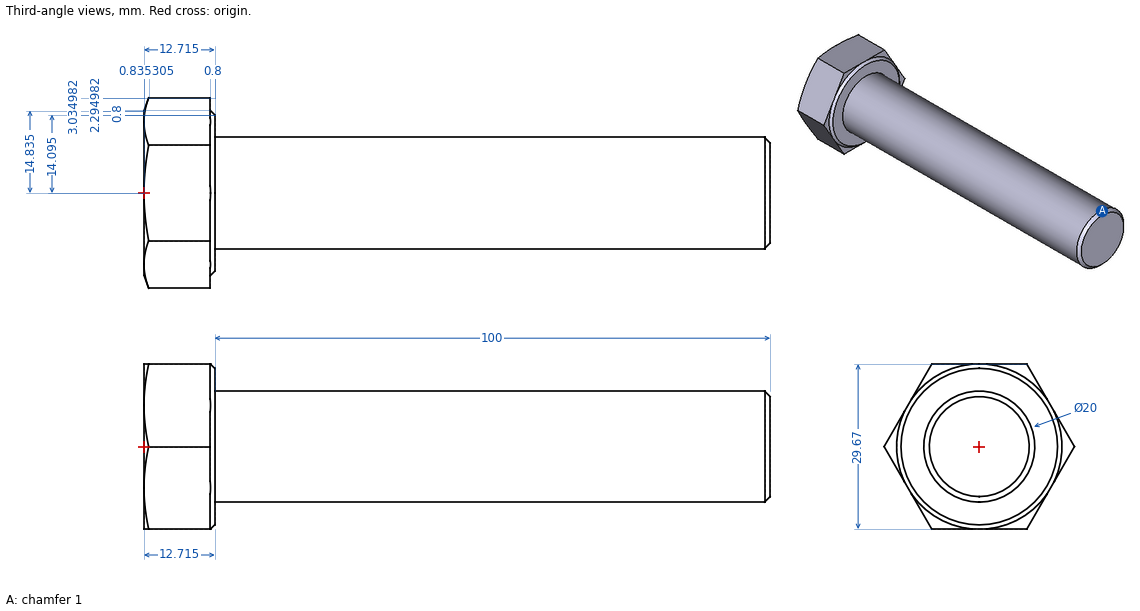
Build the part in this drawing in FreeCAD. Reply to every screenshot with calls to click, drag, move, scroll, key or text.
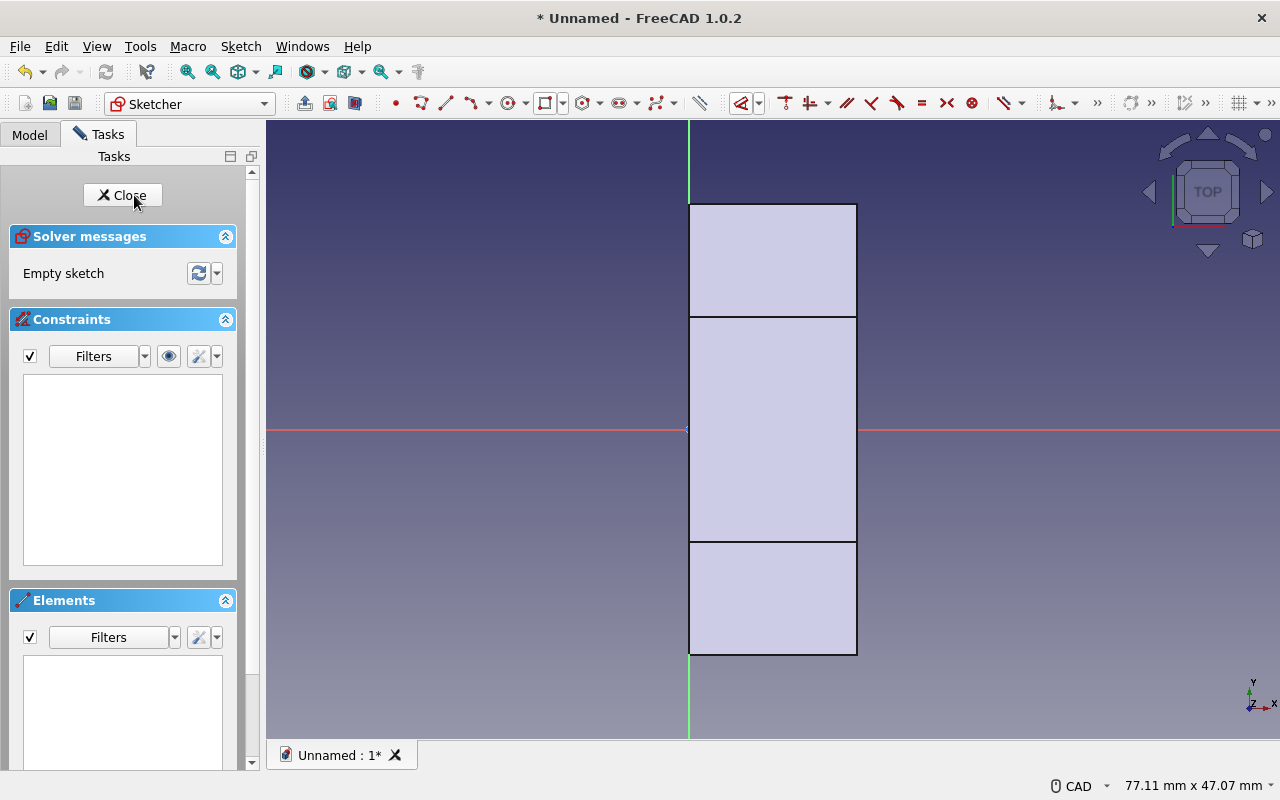
key(q)
key(s)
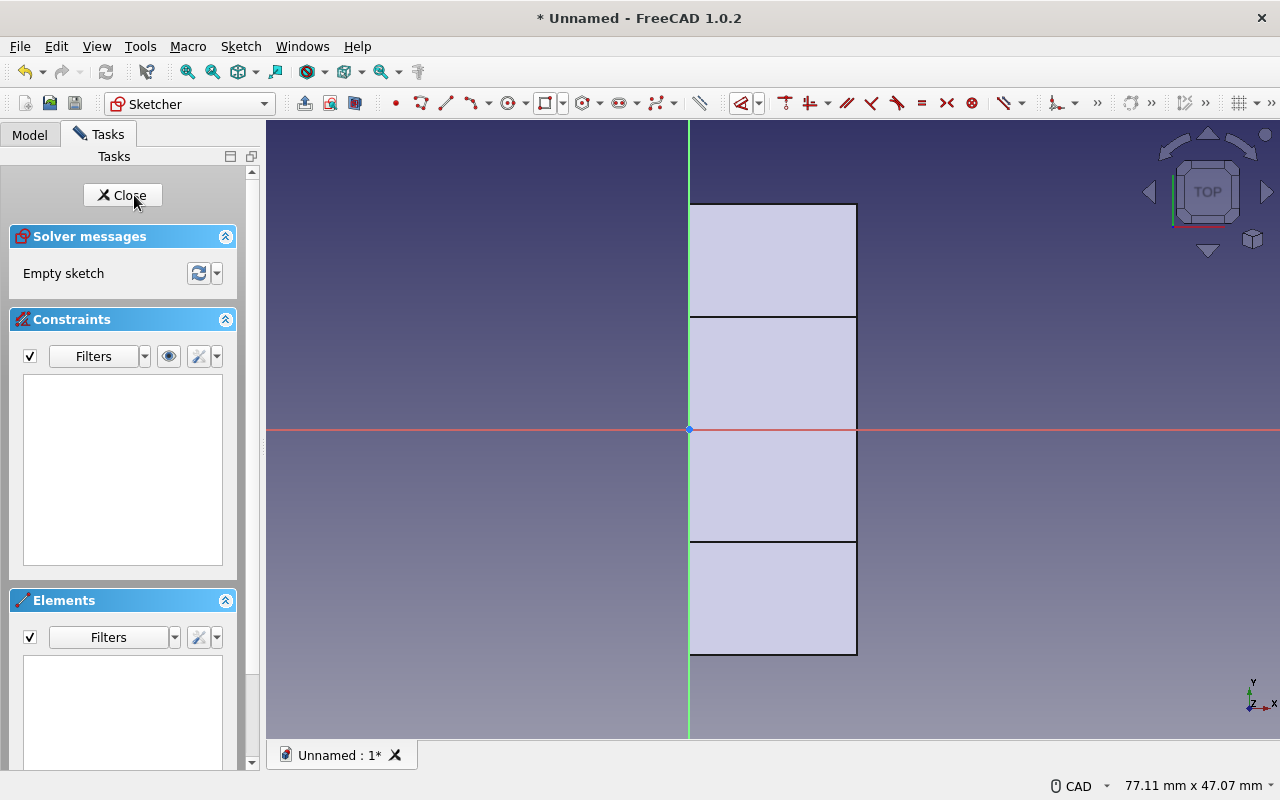
scroll(870, 199, up, 11)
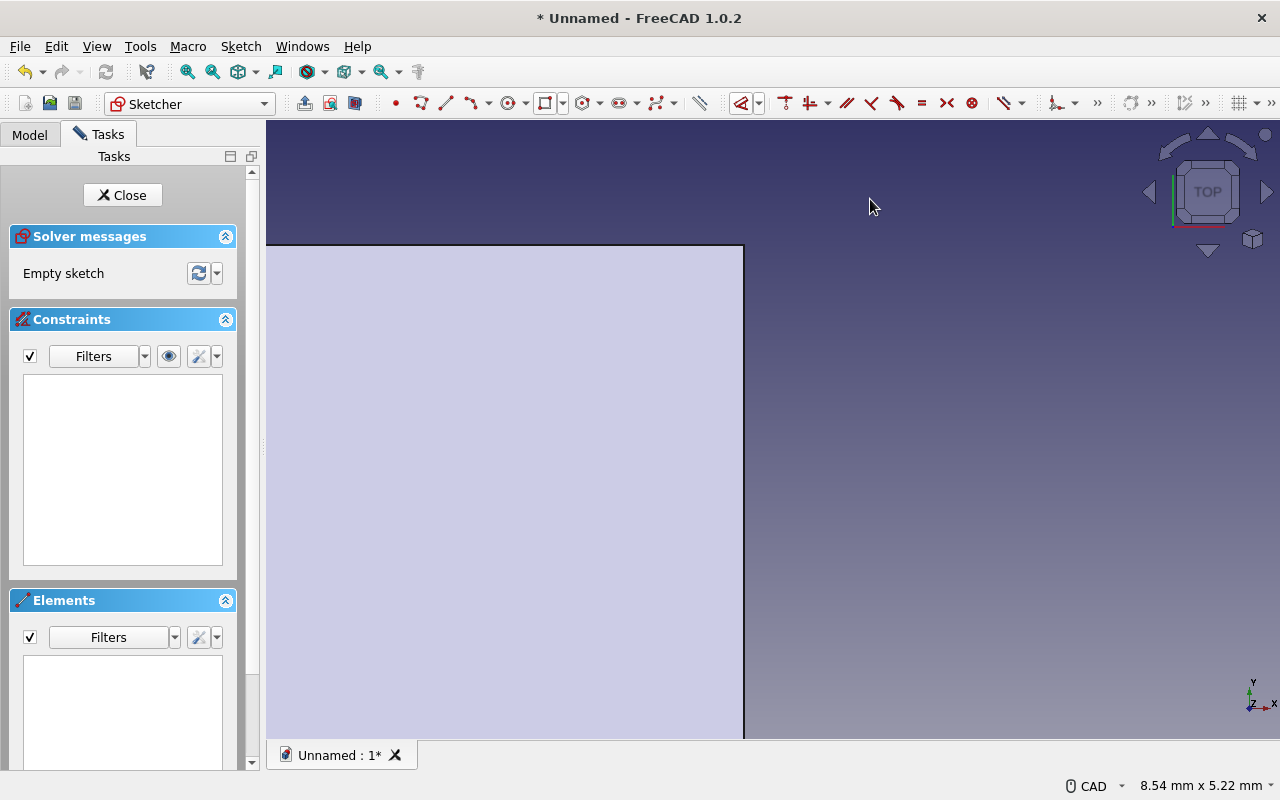
key(g)
key(m)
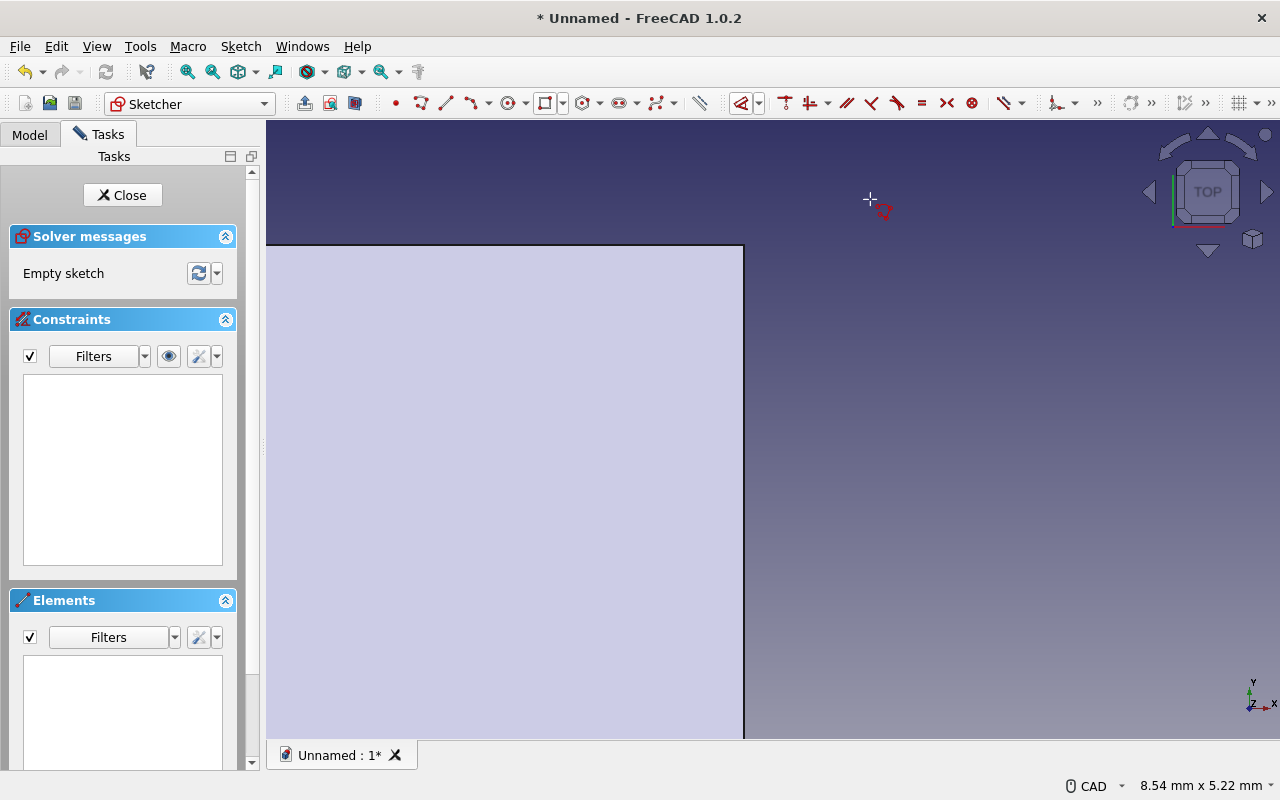
click(744, 605)
click(744, 245)
click(649, 245)
click(649, 510)
click(744, 606)
key(Escape)
key(Escape)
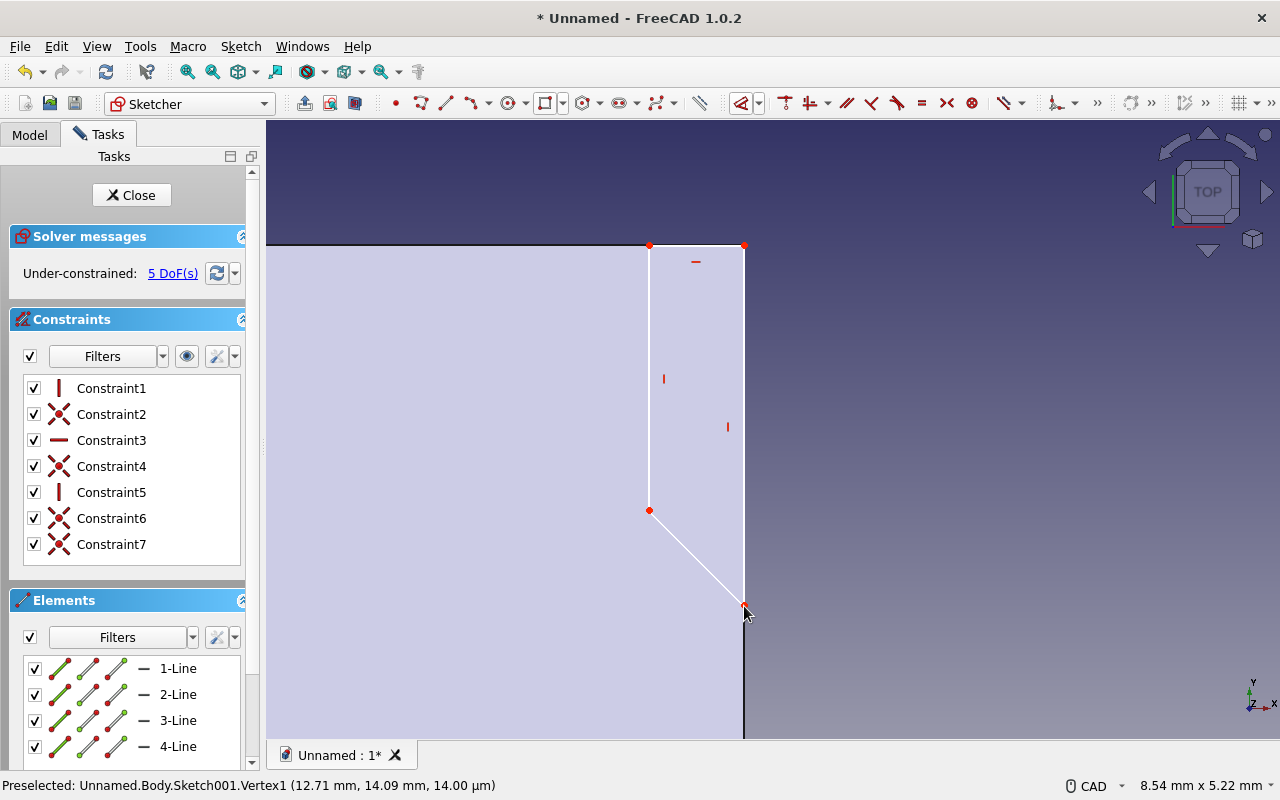
key(d)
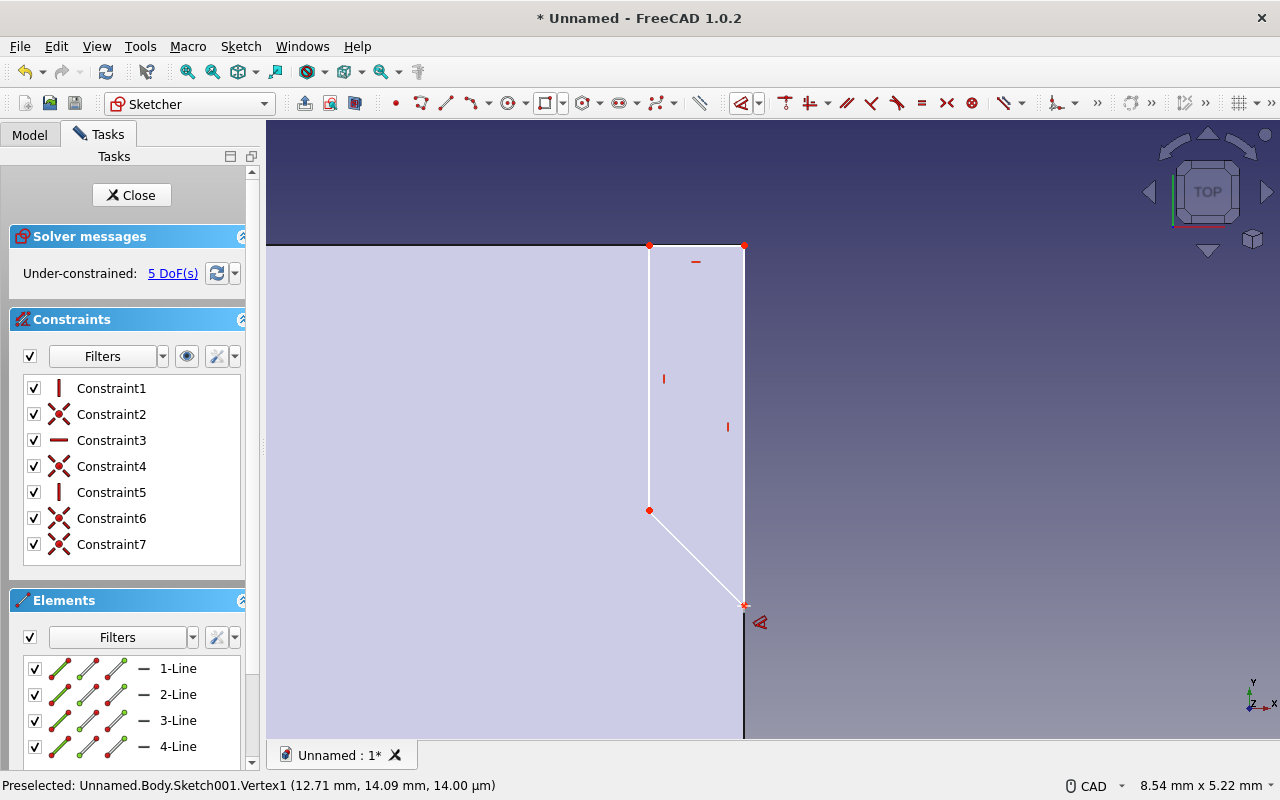
click(715, 246)
click(696, 212)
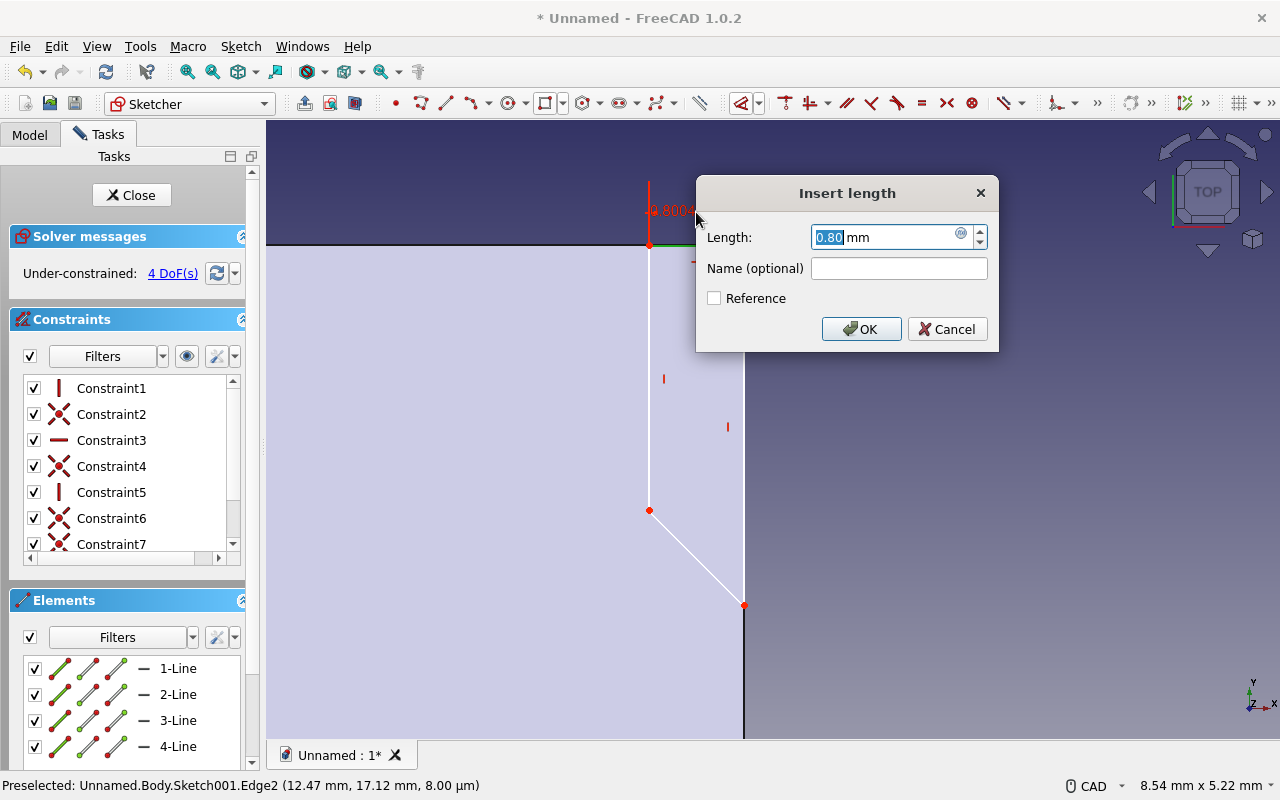
text(0.8)
key(Return)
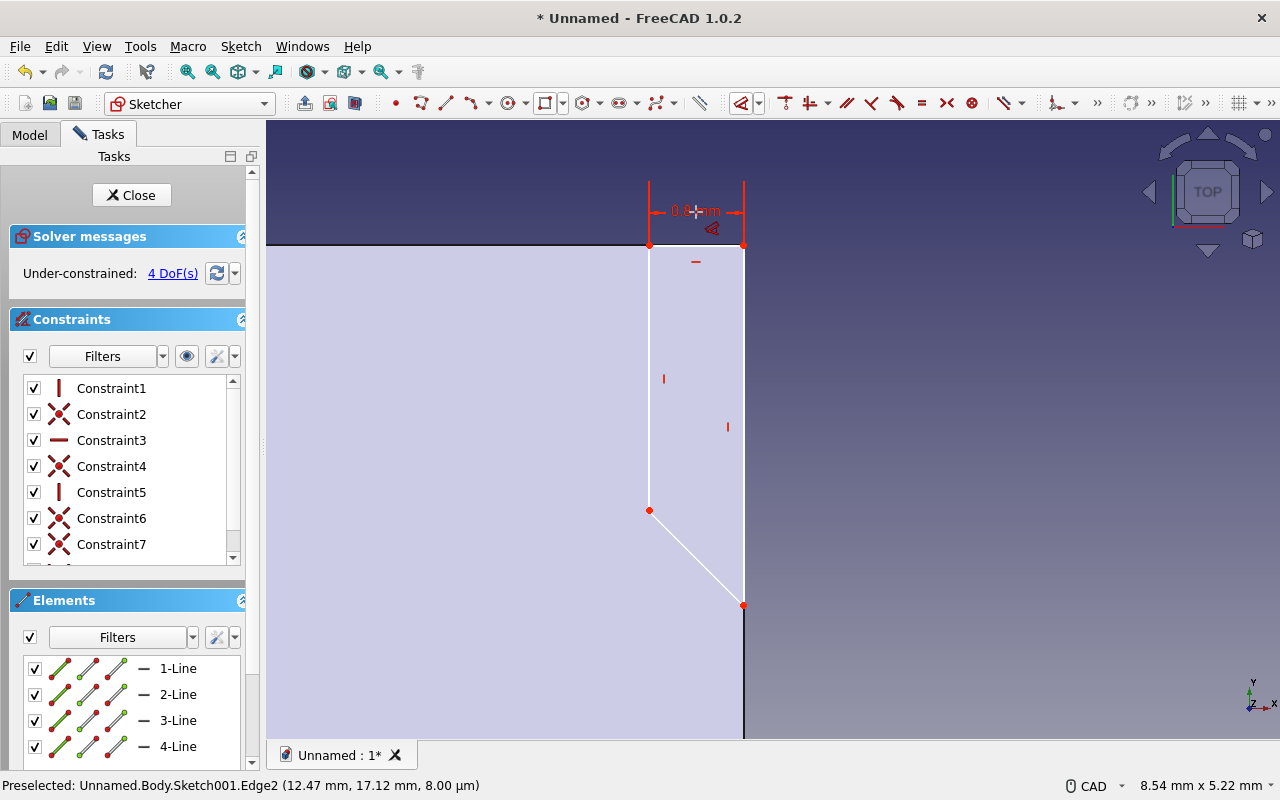
click(677, 539)
click(615, 558)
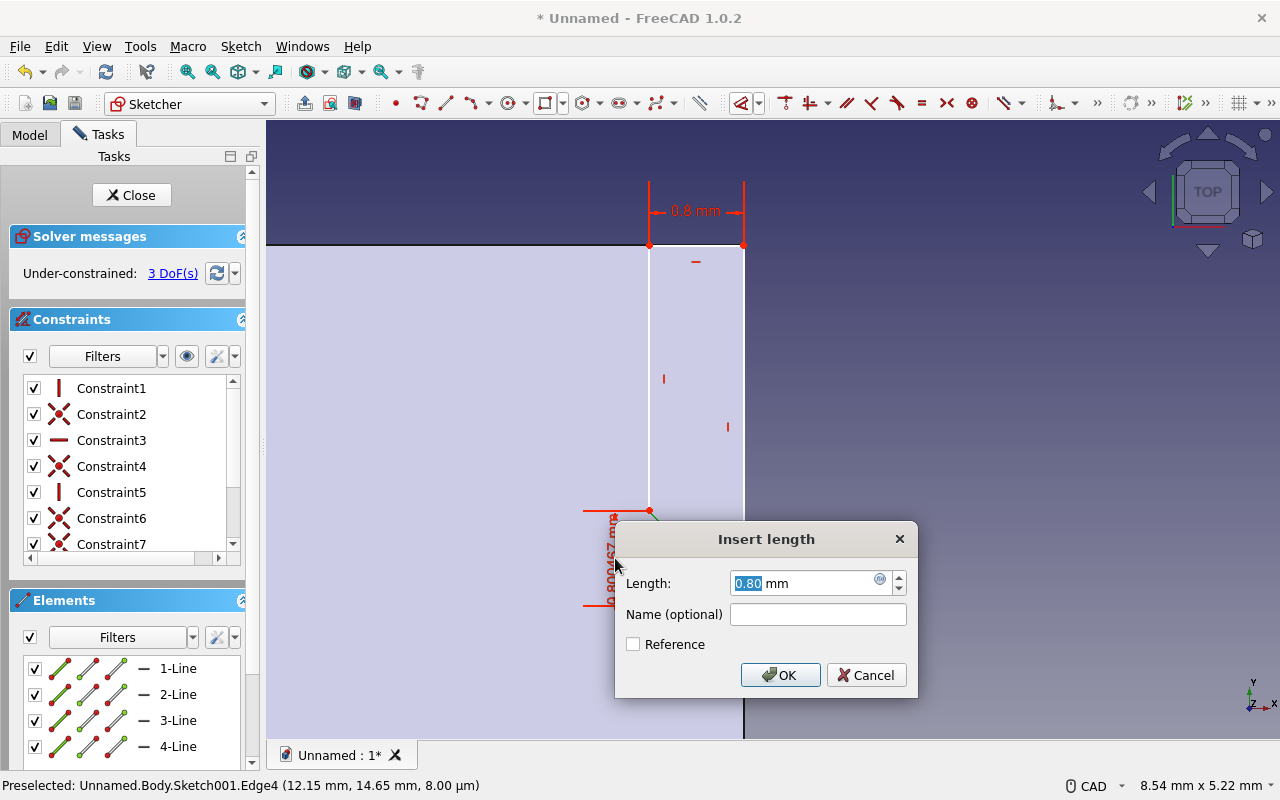
text(0.8)
key(Return)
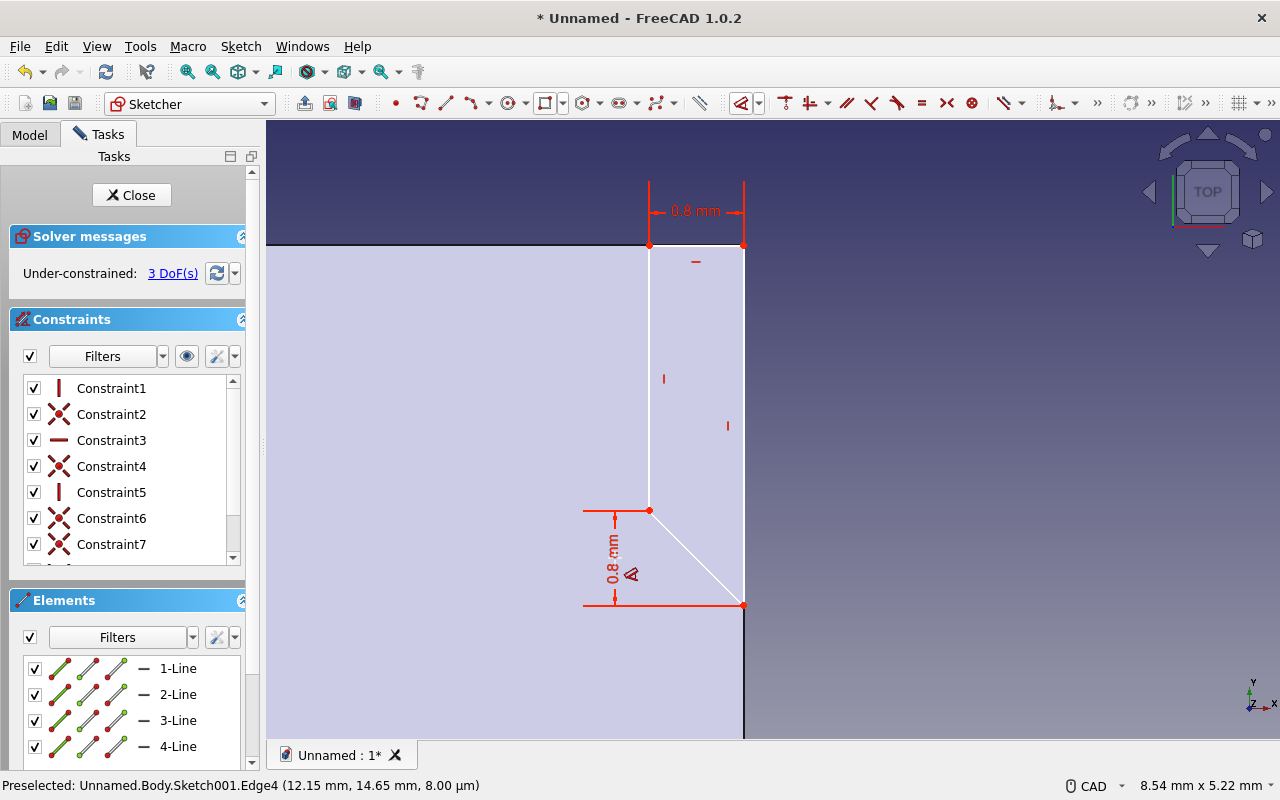
click(744, 606)
click(519, 572)